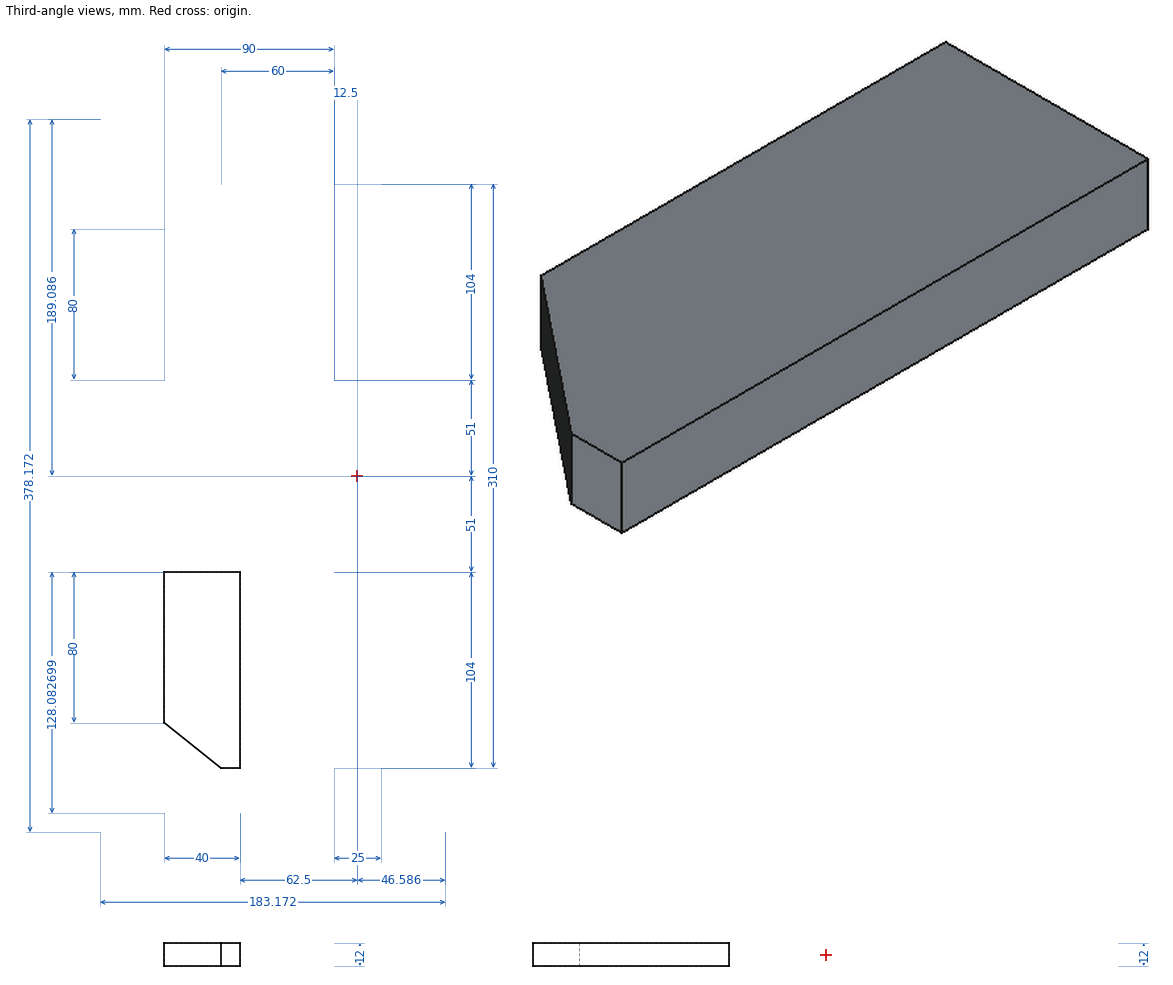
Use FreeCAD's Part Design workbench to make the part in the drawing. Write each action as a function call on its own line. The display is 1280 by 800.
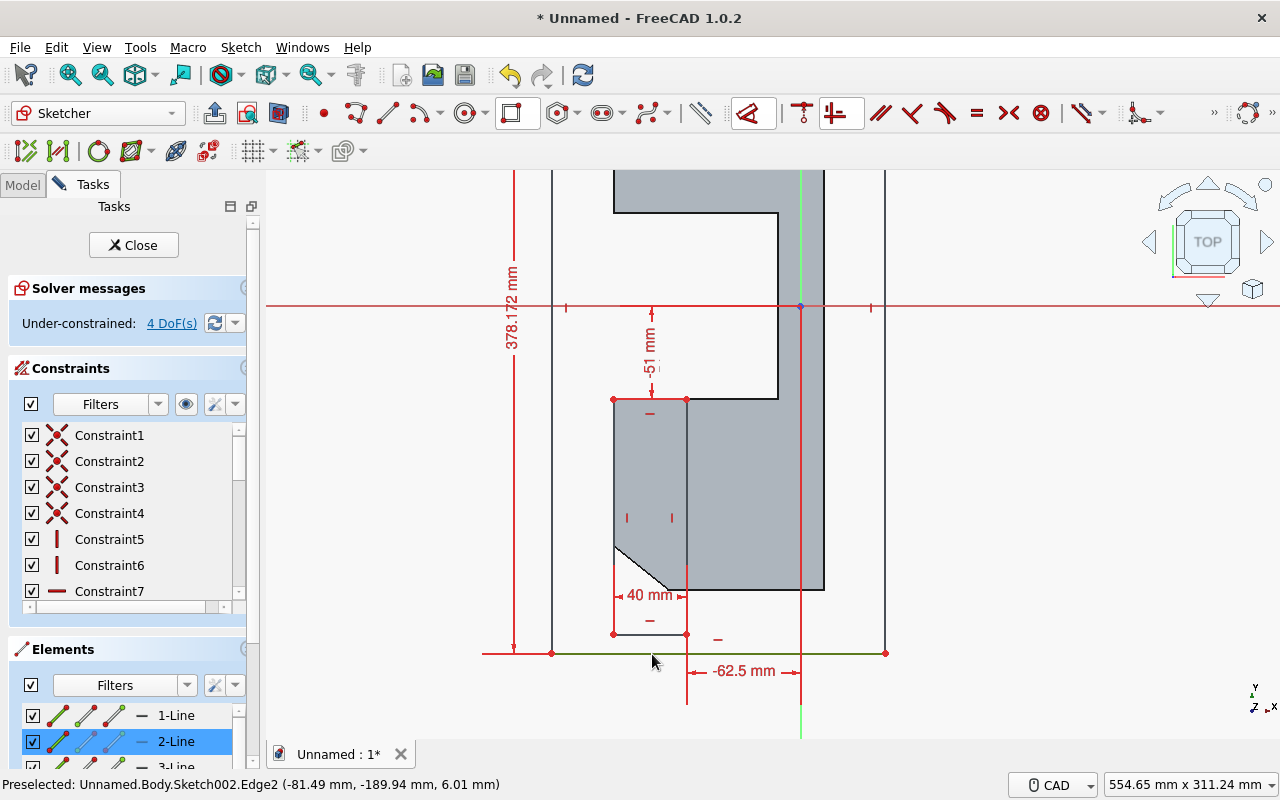
click(770, 114)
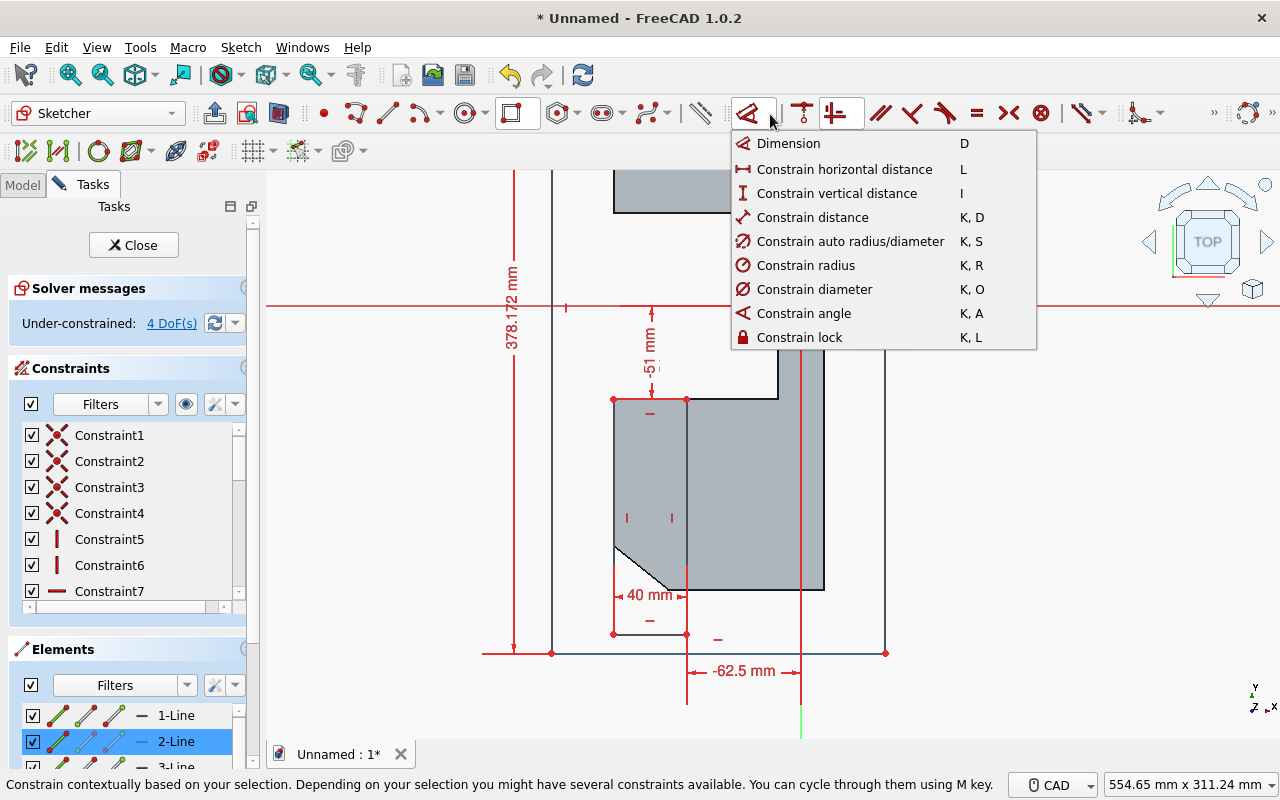
click(884, 169)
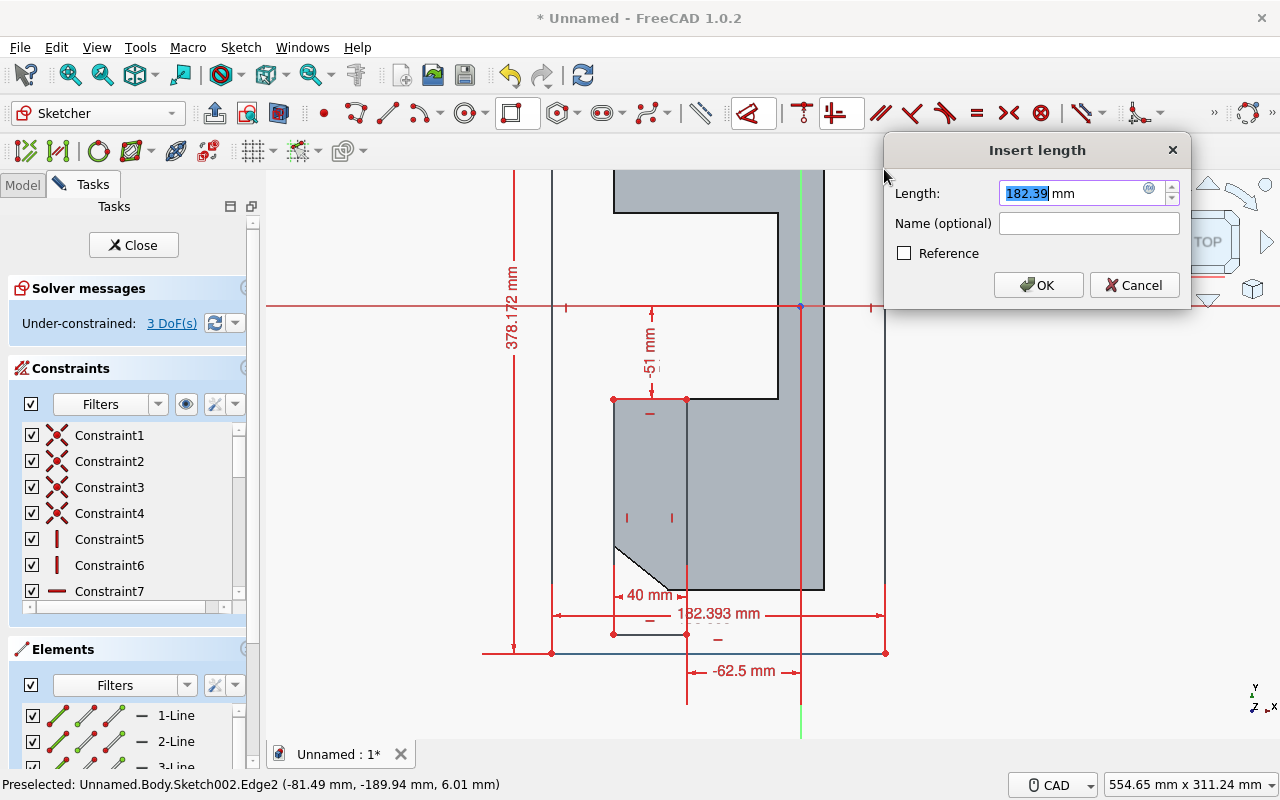
text(183.172)
key(Return)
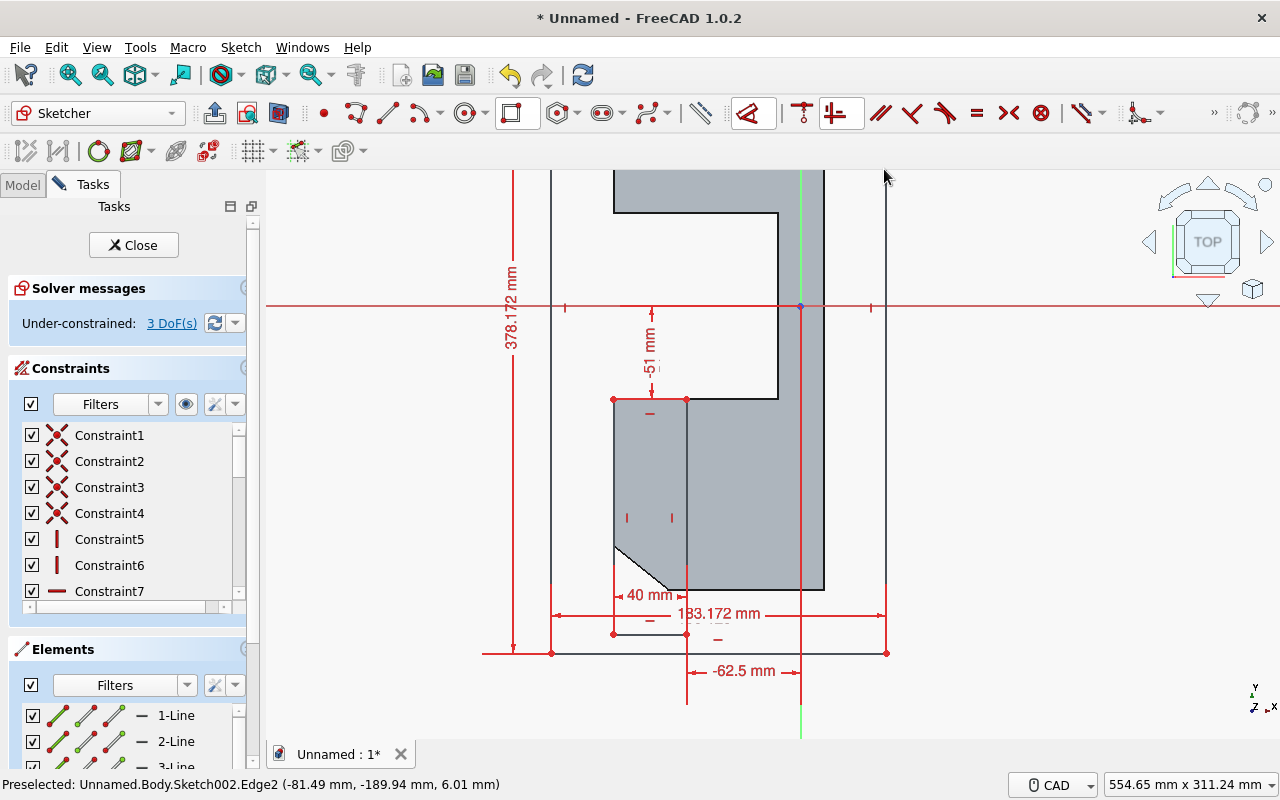
click(886, 654)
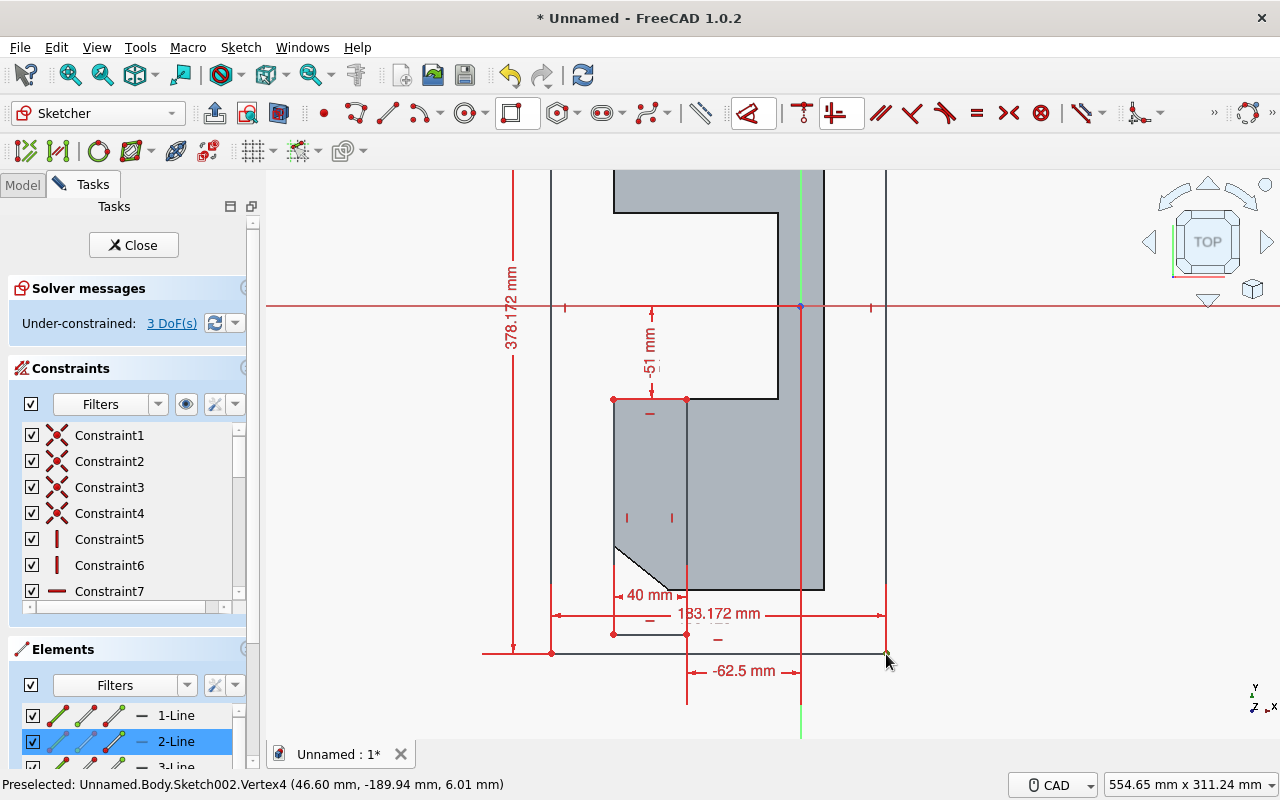
key(l)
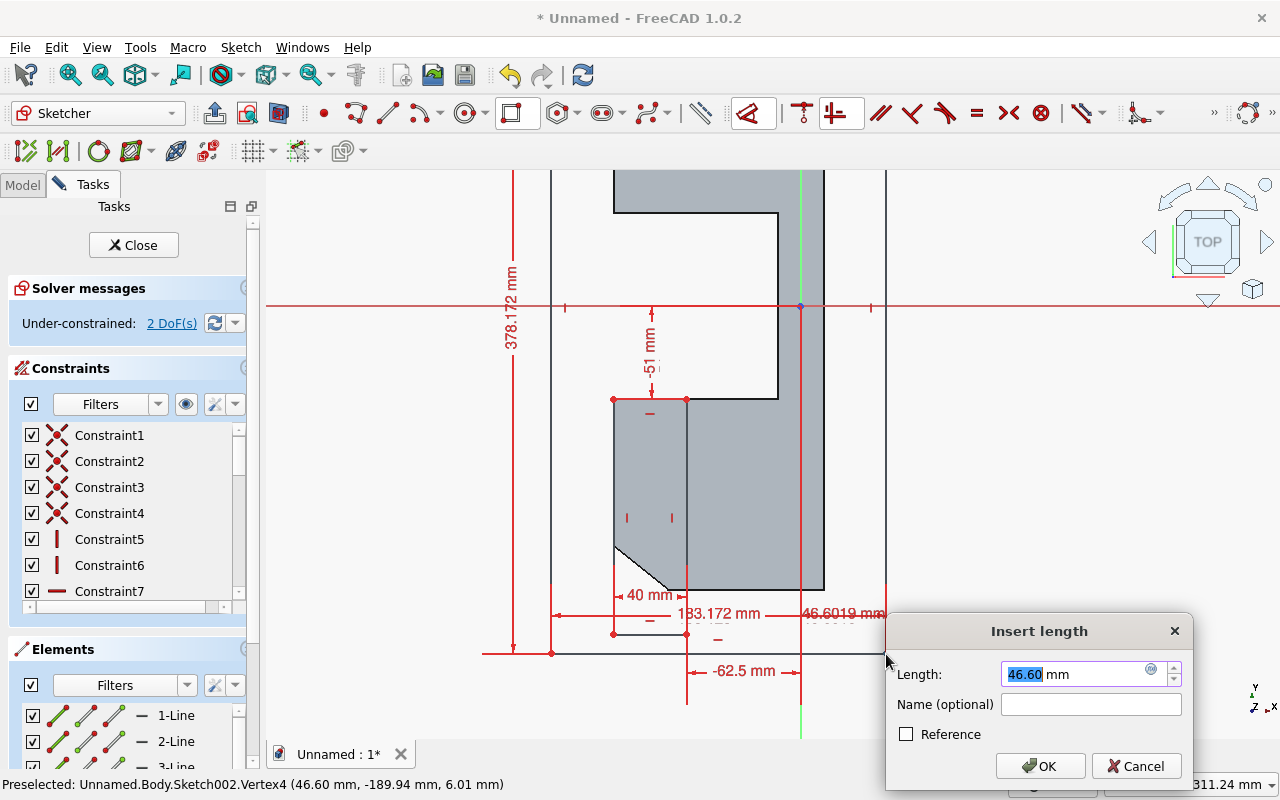
text(46.586)
key(Return)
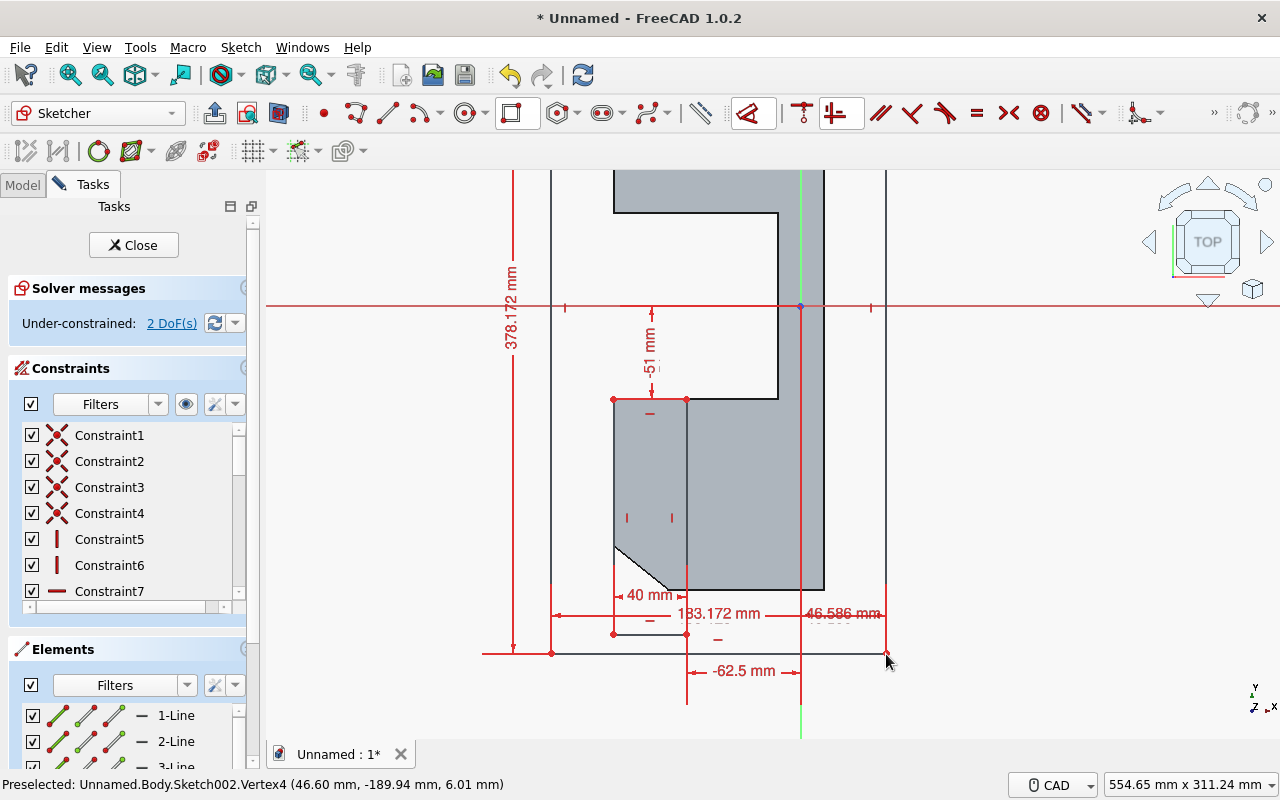
scroll(687, 635, down, 3)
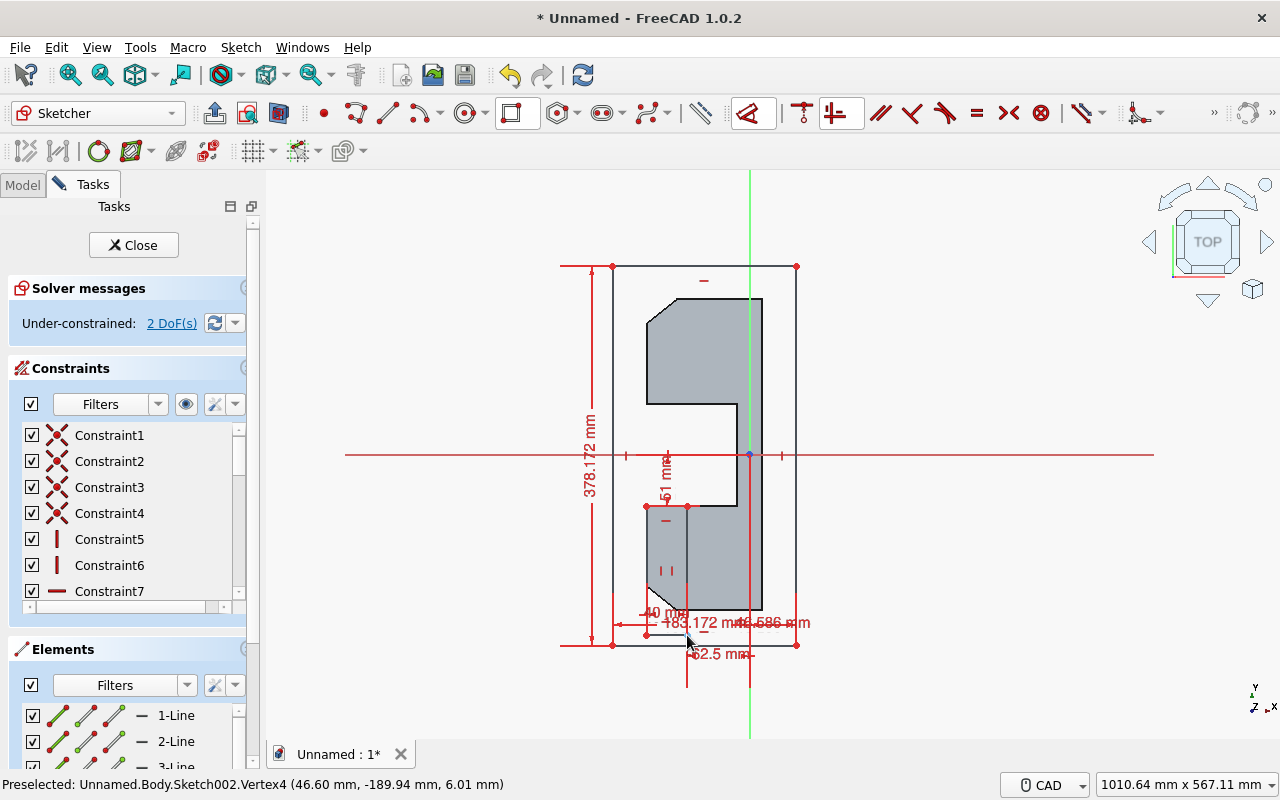
click(613, 266)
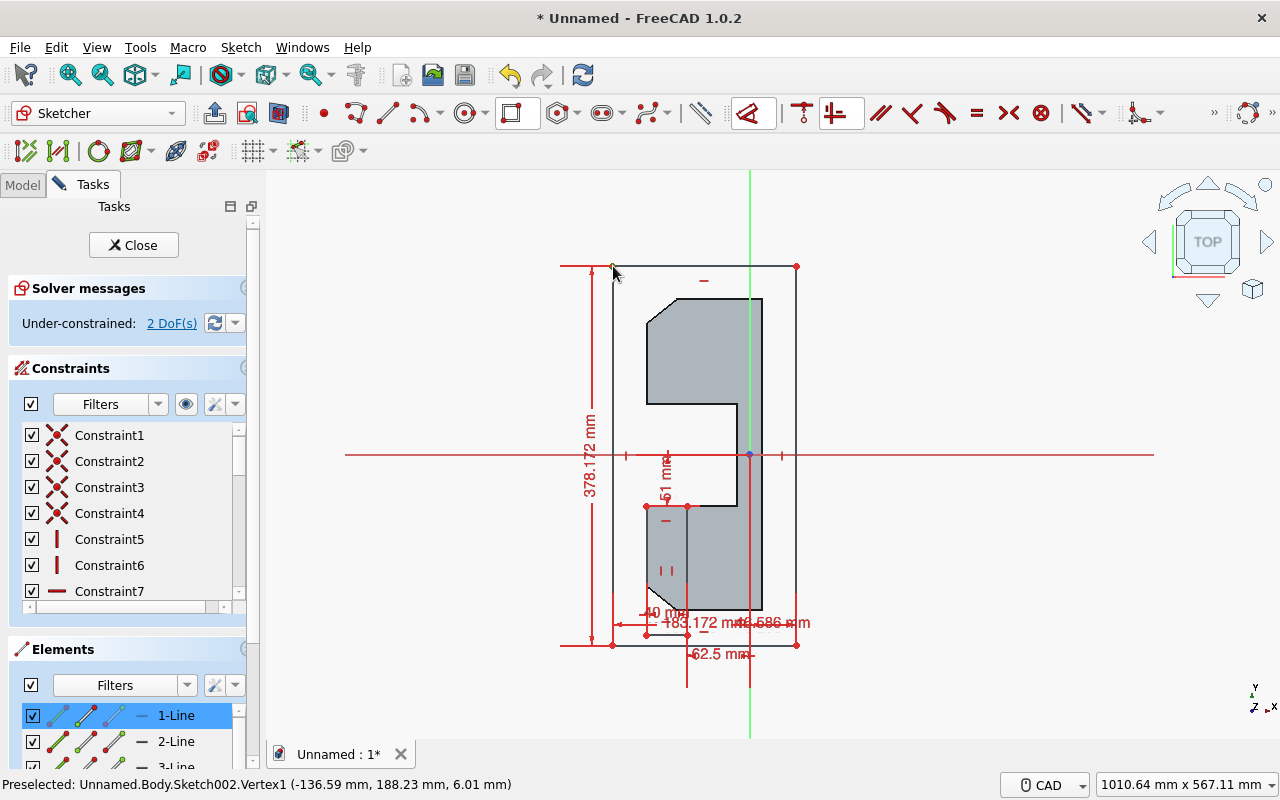
click(770, 114)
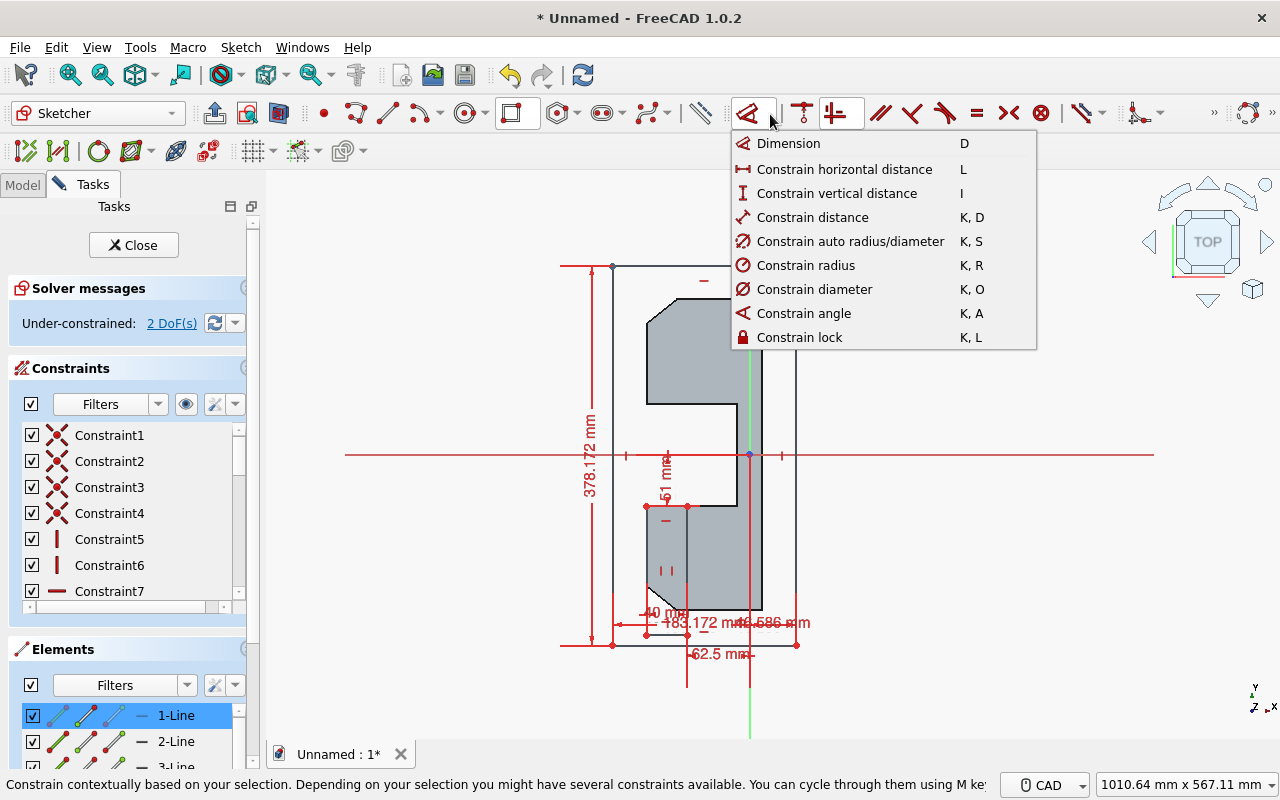
click(884, 193)